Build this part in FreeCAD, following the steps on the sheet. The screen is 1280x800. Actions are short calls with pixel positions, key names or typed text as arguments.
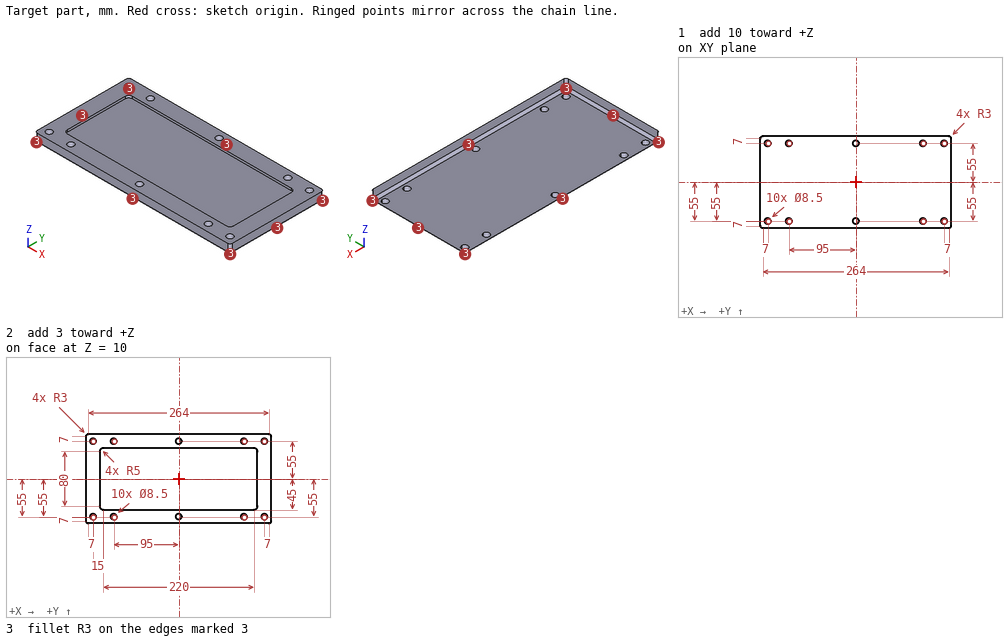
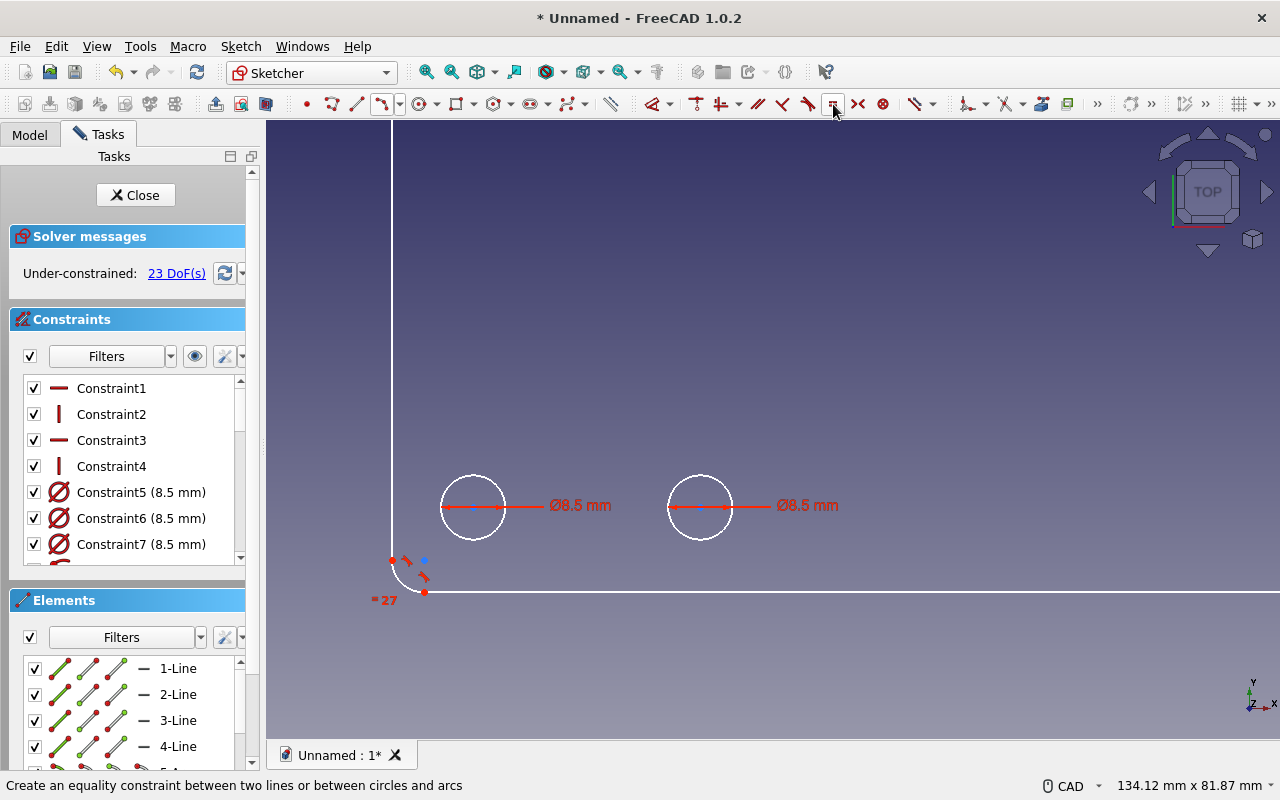
click(700, 507)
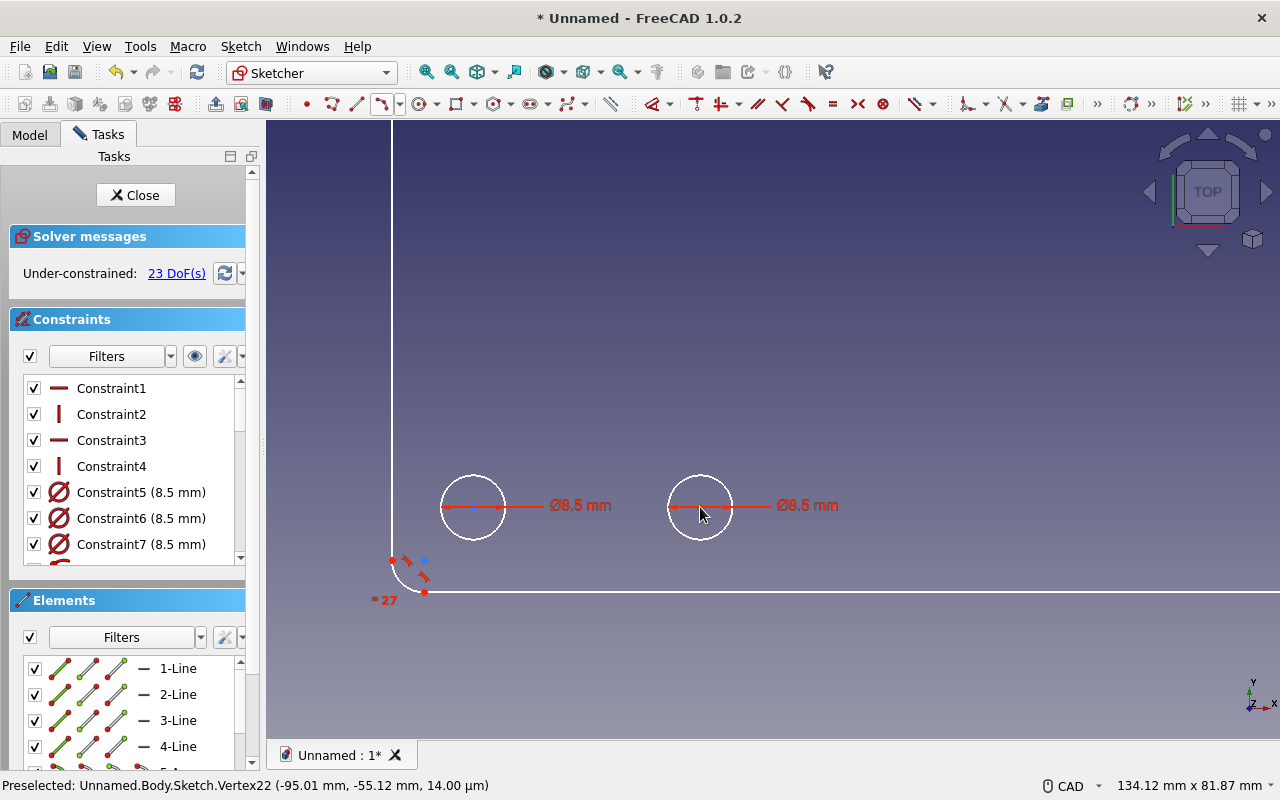
scroll(397, 576, down, 6)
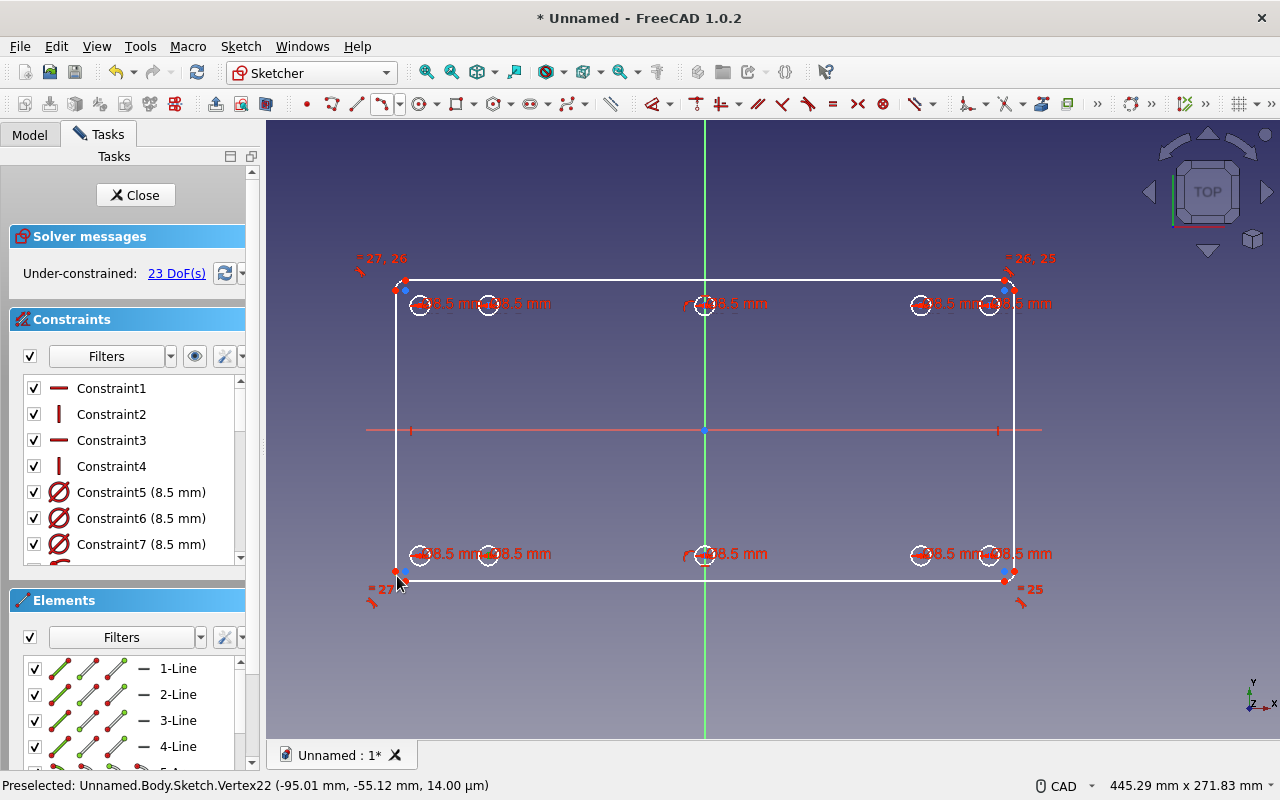
click(921, 556)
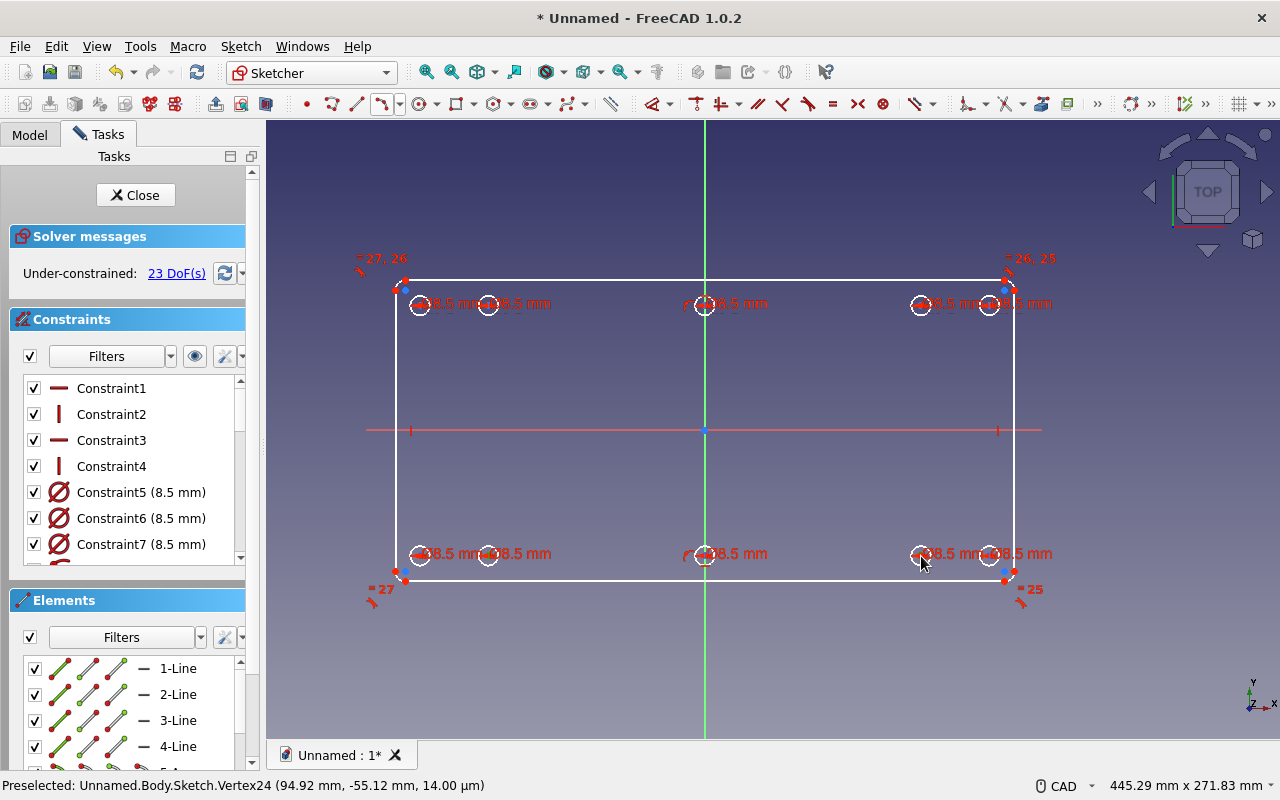
click(705, 671)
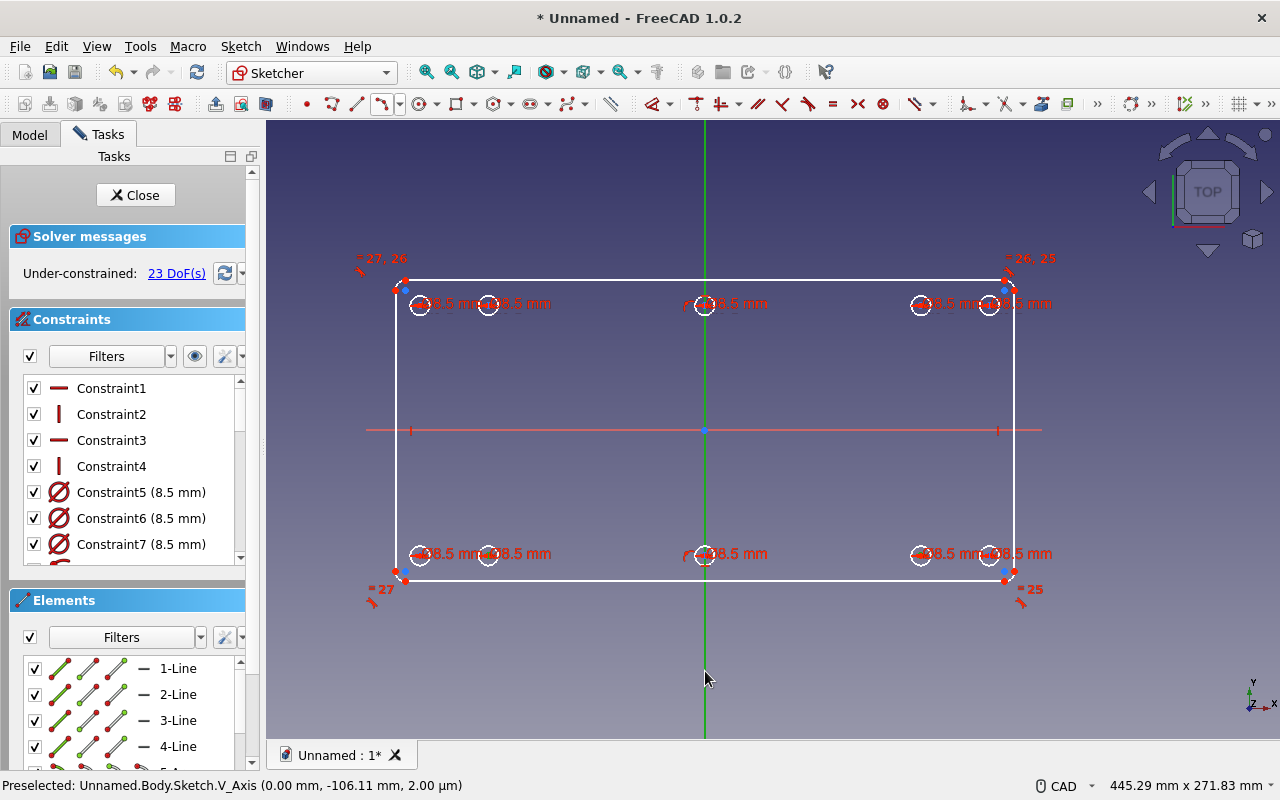
click(858, 104)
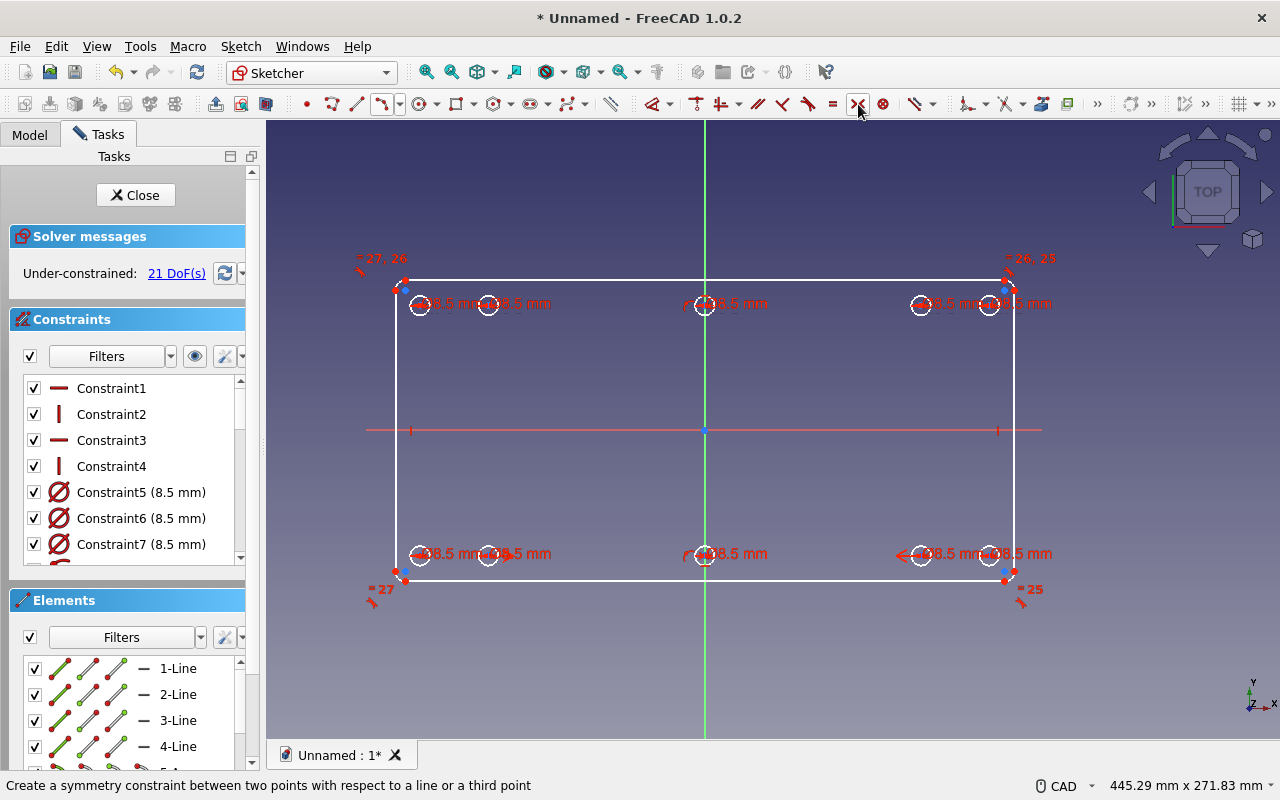
click(420, 556)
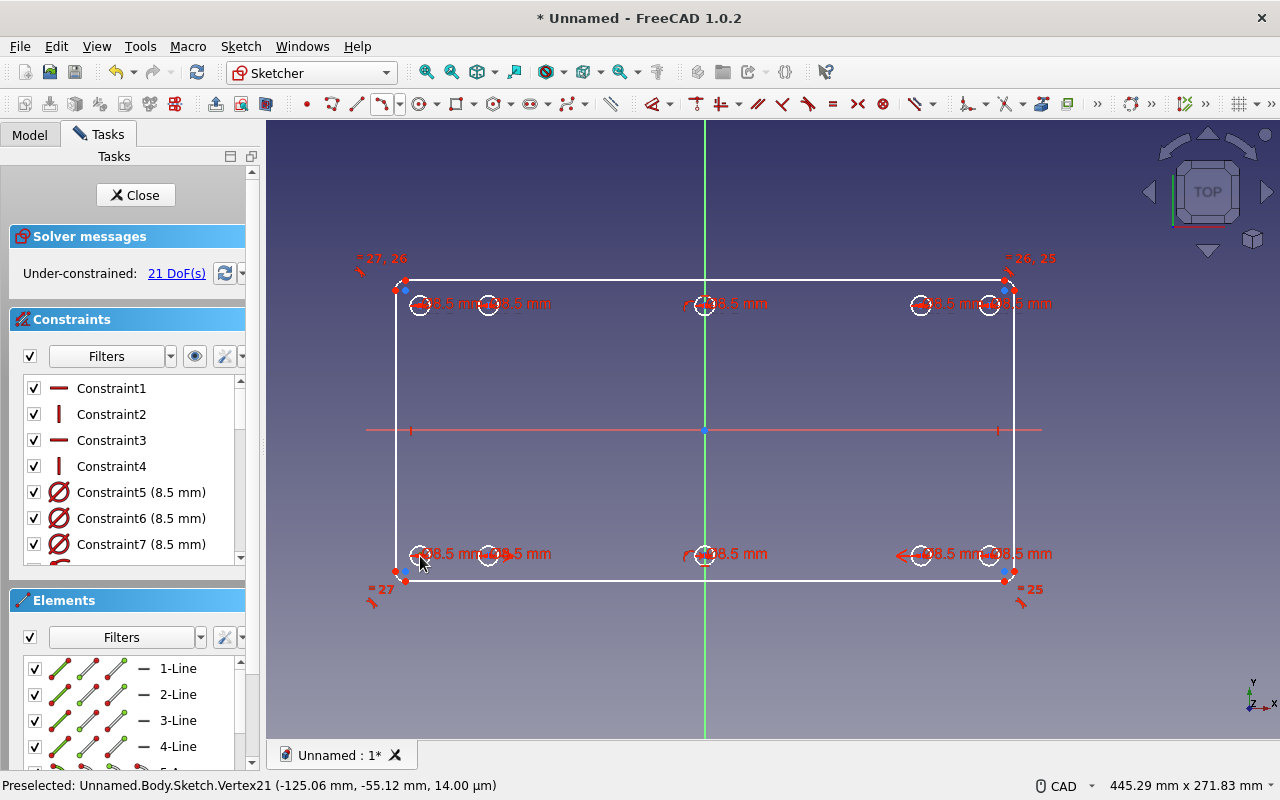
click(989, 556)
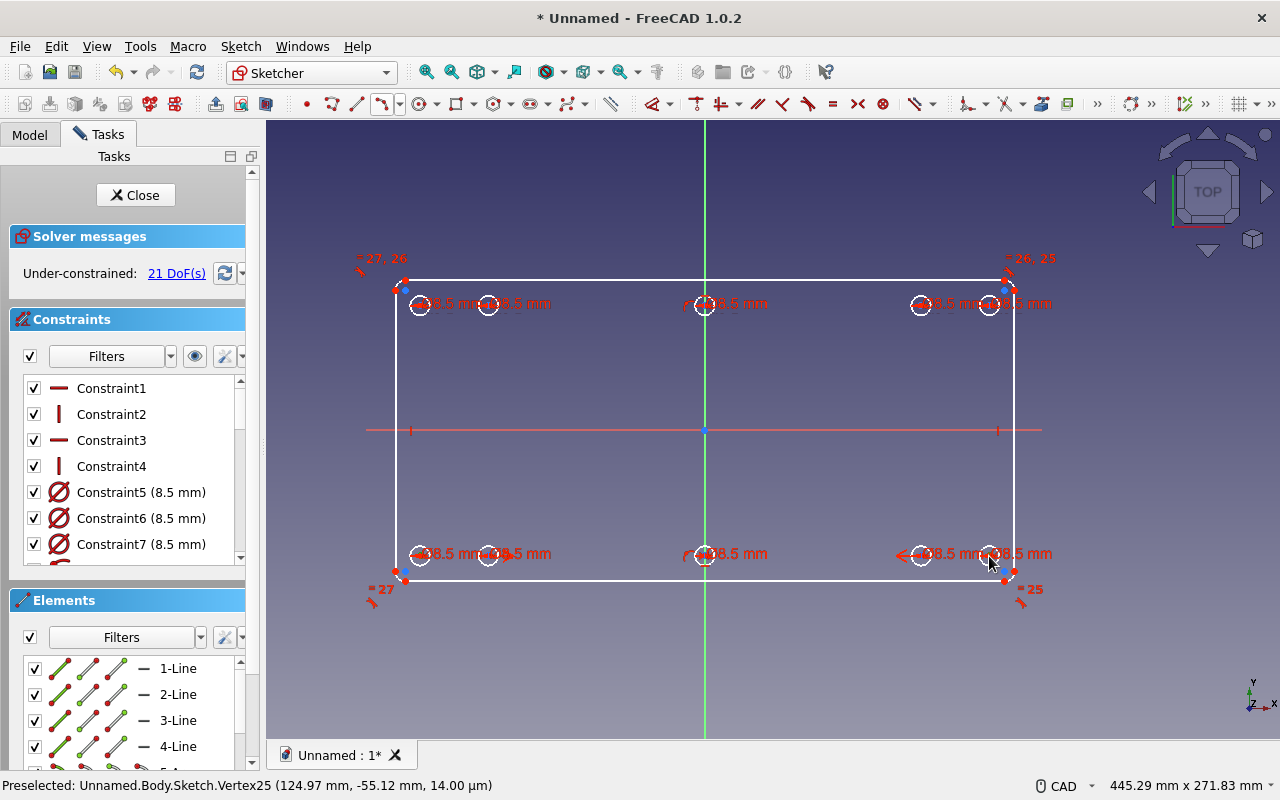
click(705, 671)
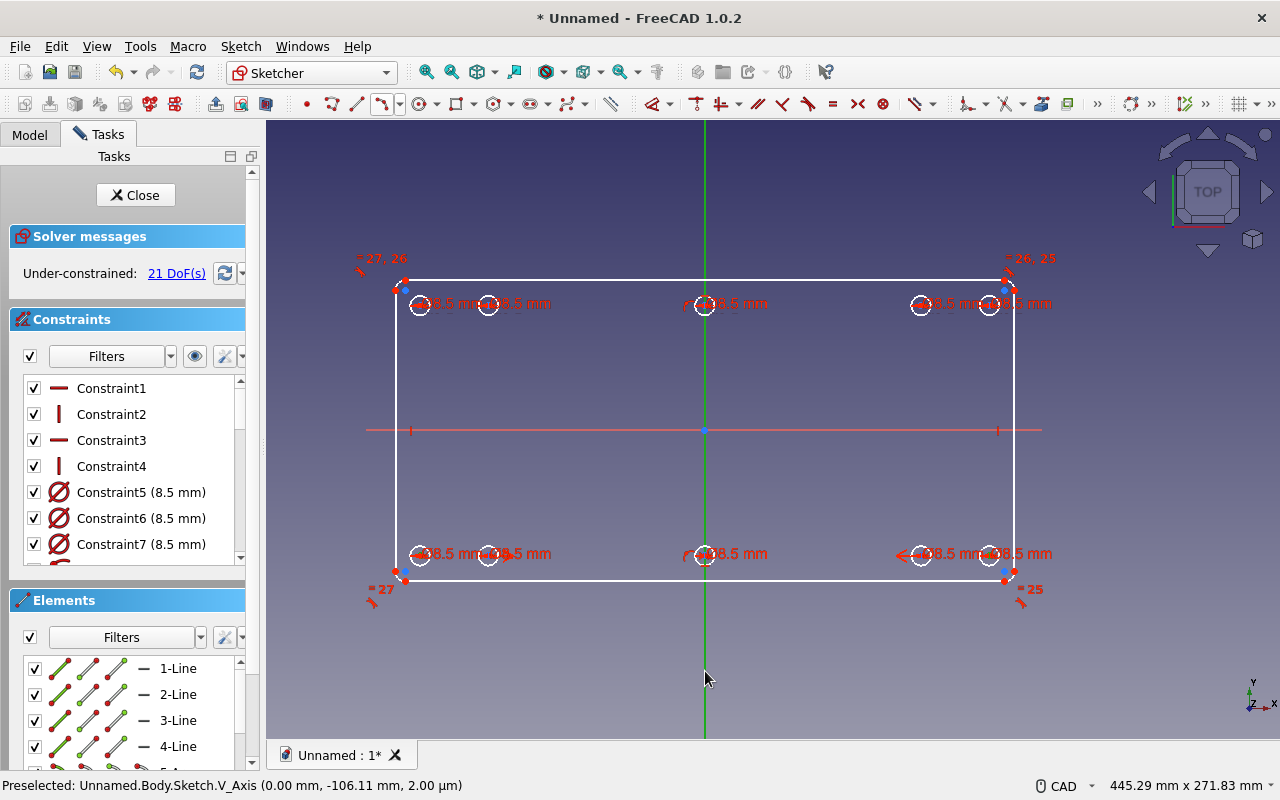
click(858, 104)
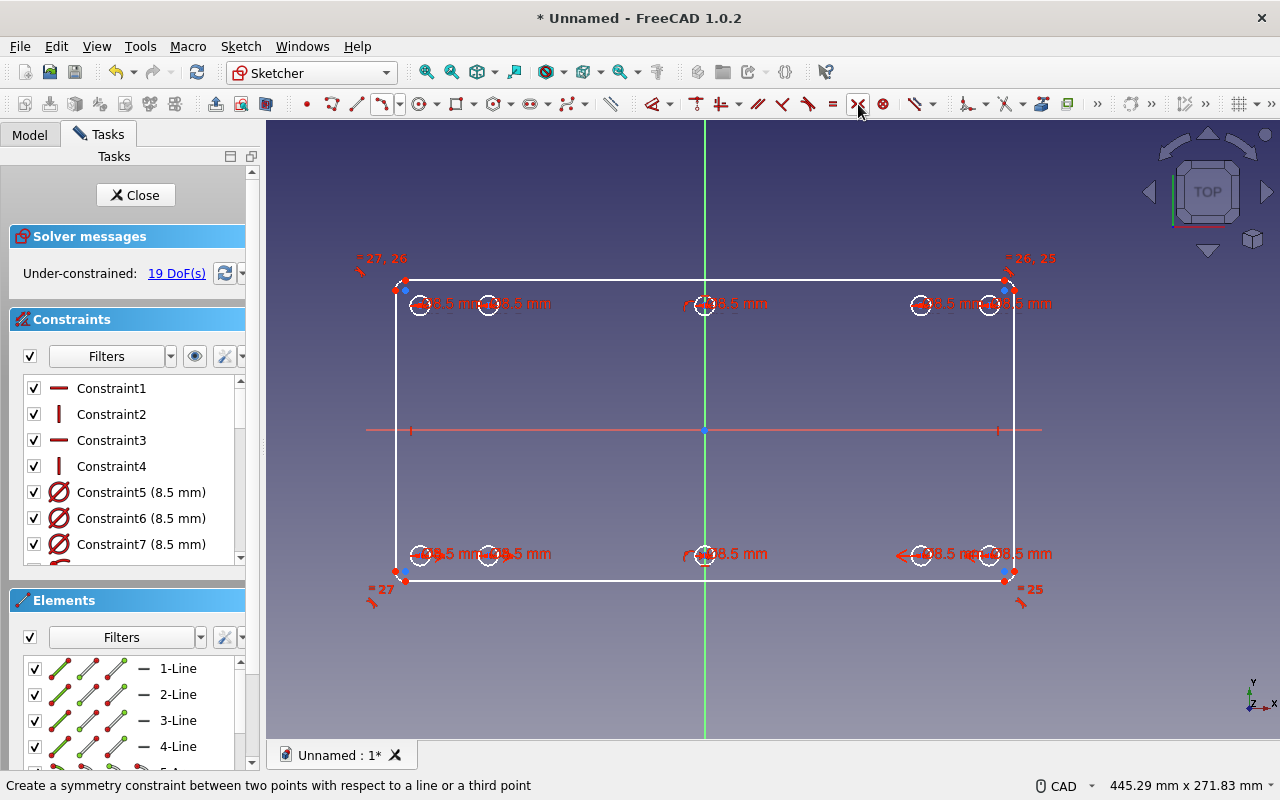
click(420, 556)